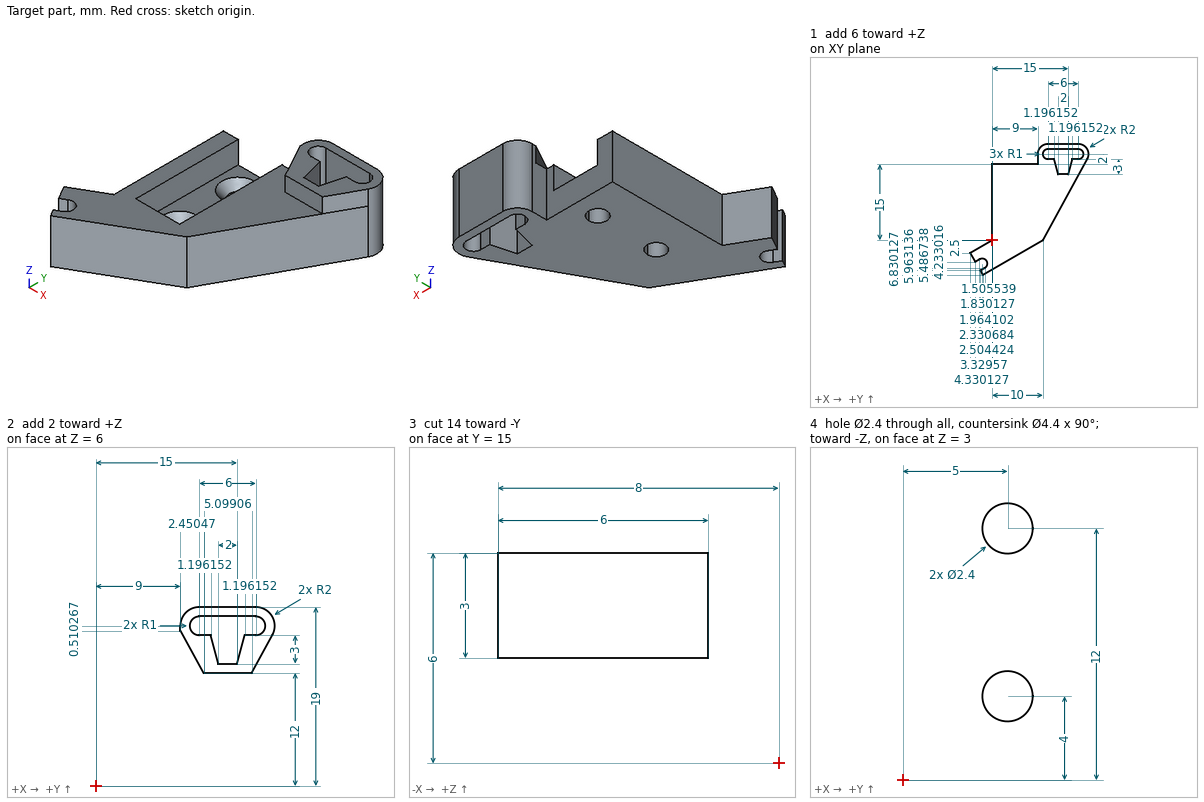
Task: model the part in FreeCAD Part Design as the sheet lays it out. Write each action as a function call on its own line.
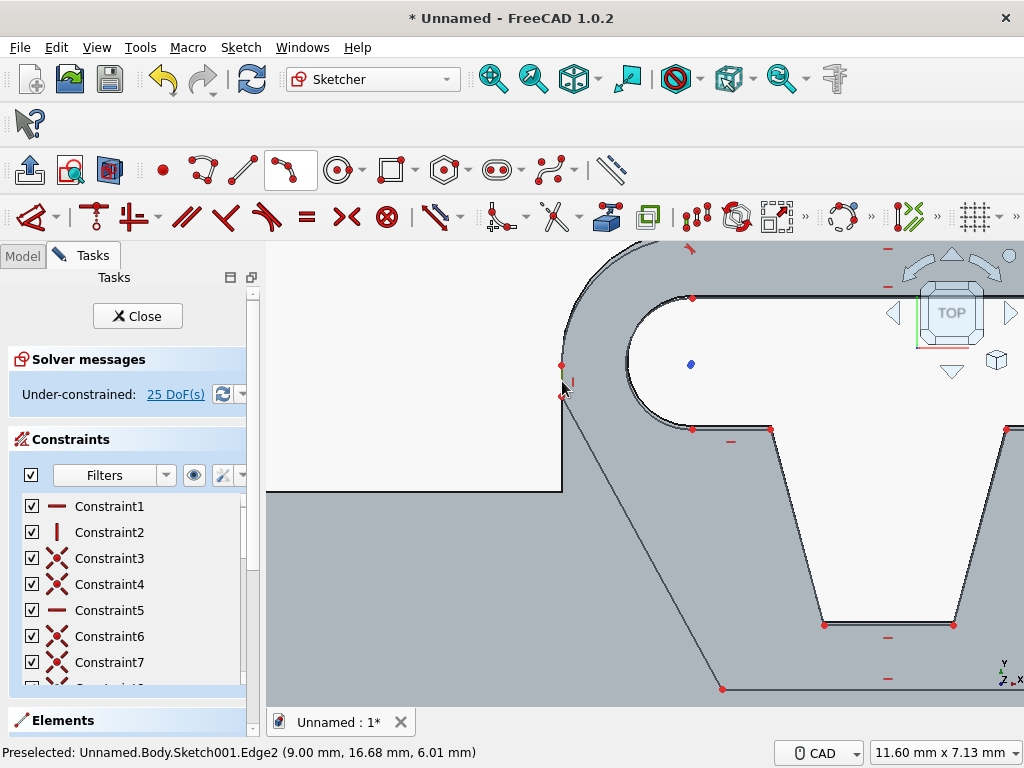
scroll(573, 351, down, 7)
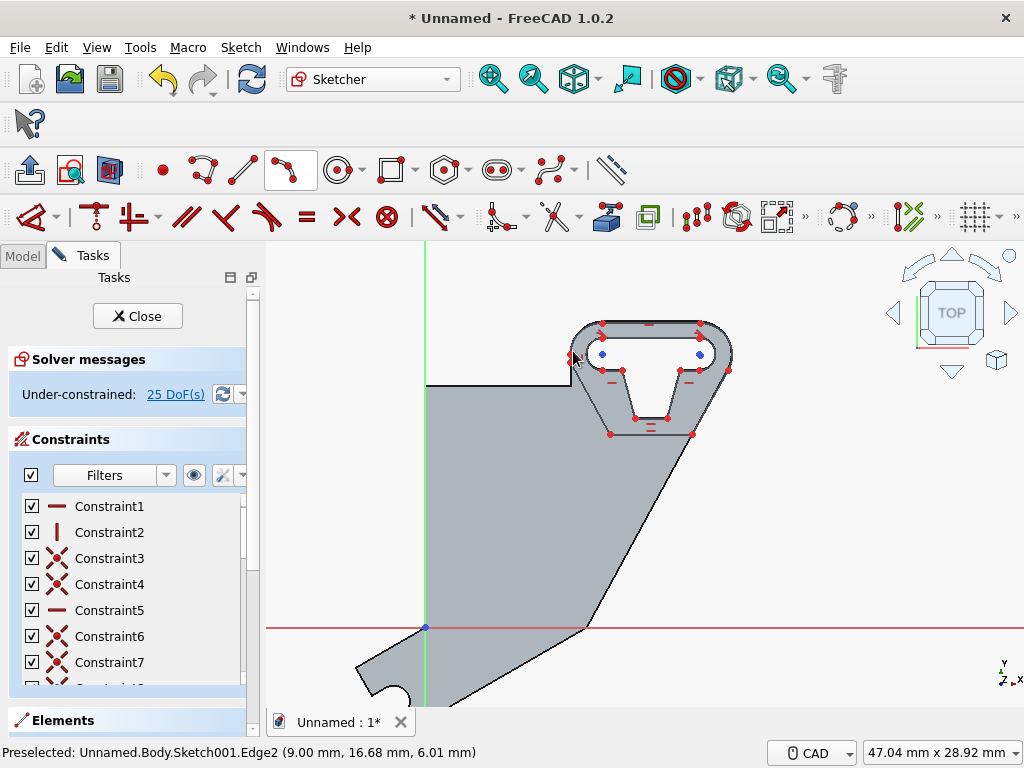
click(574, 340)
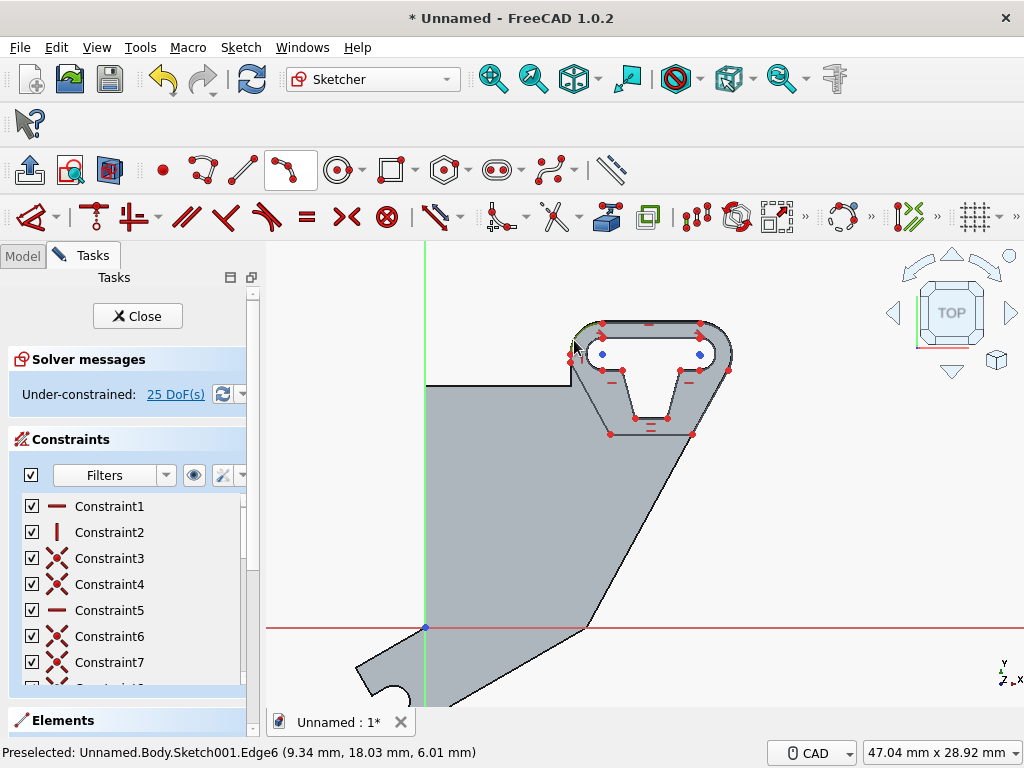
key(t)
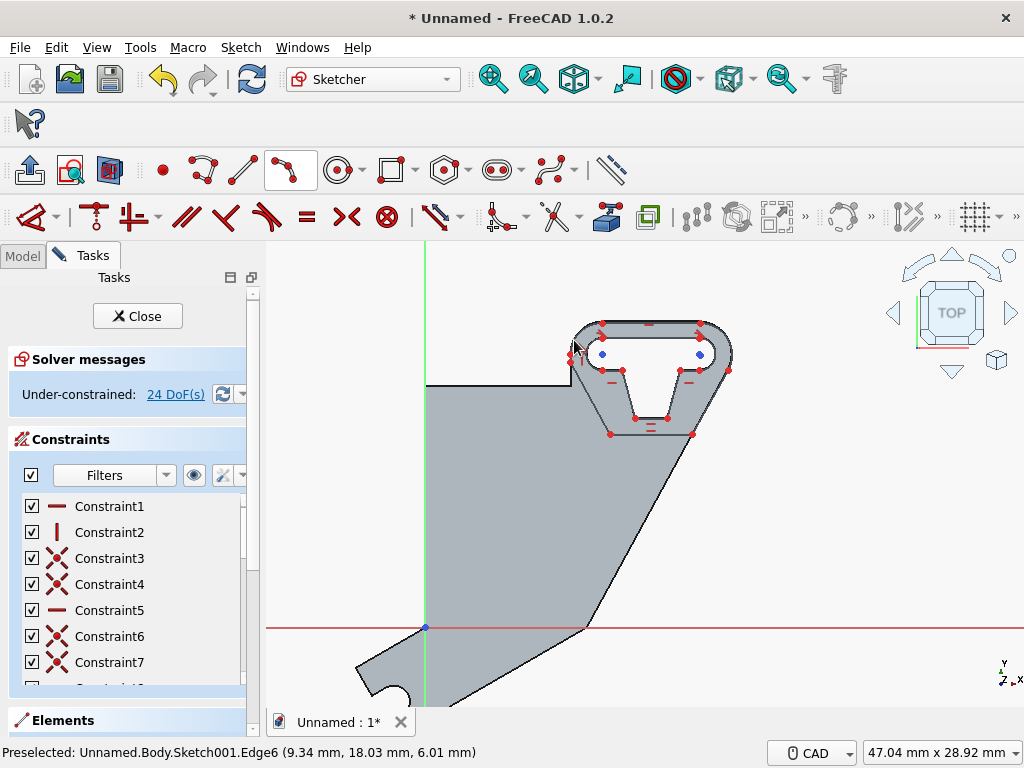
click(703, 415)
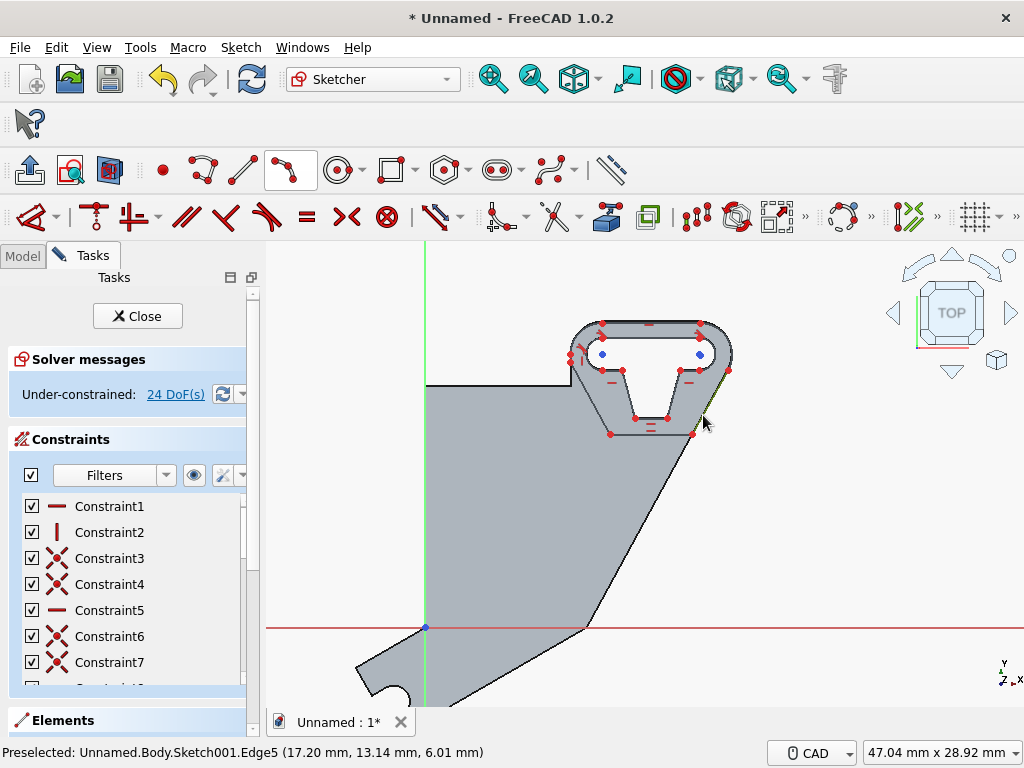
click(732, 351)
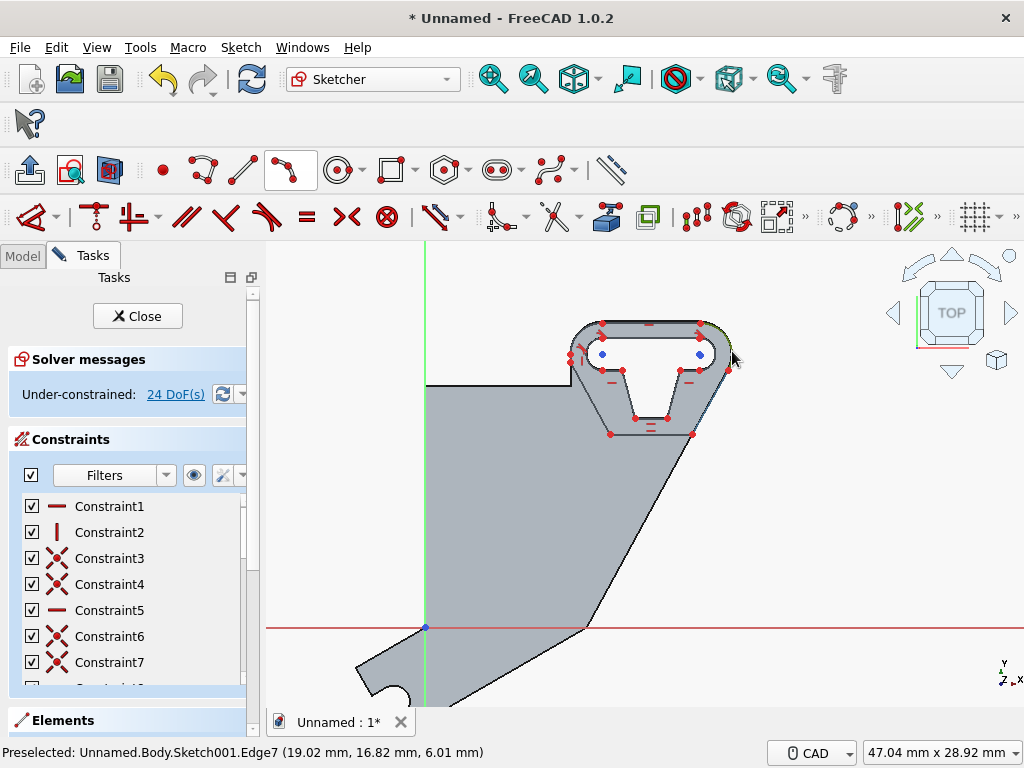
key(t)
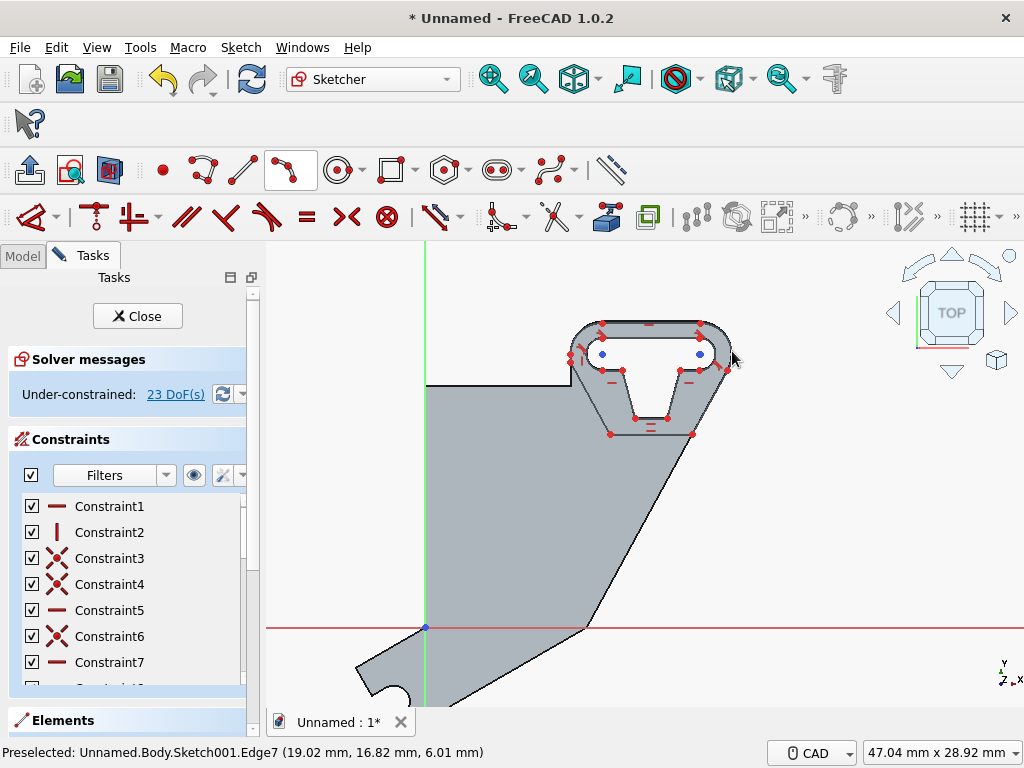
click(632, 338)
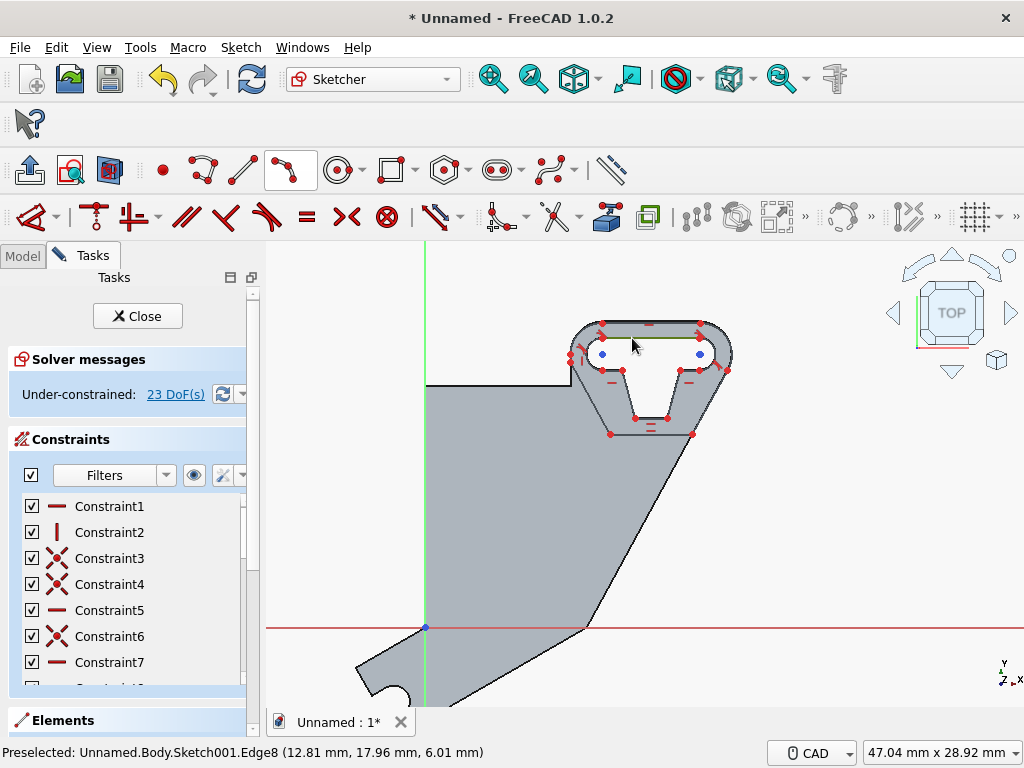
click(712, 345)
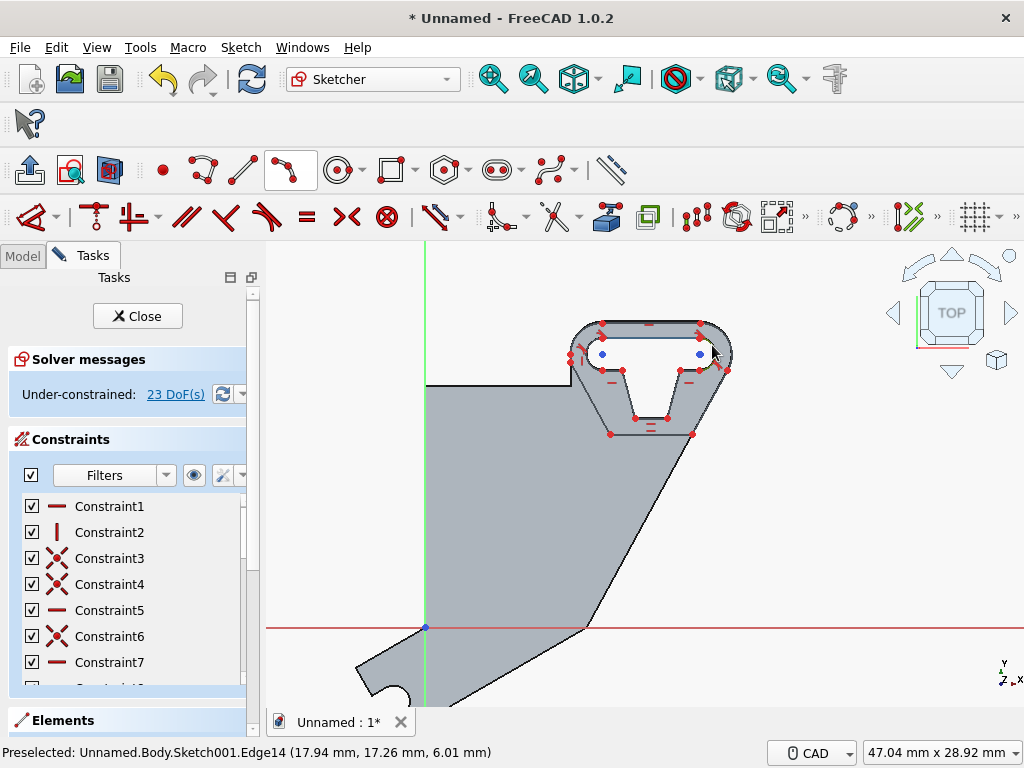
key(t)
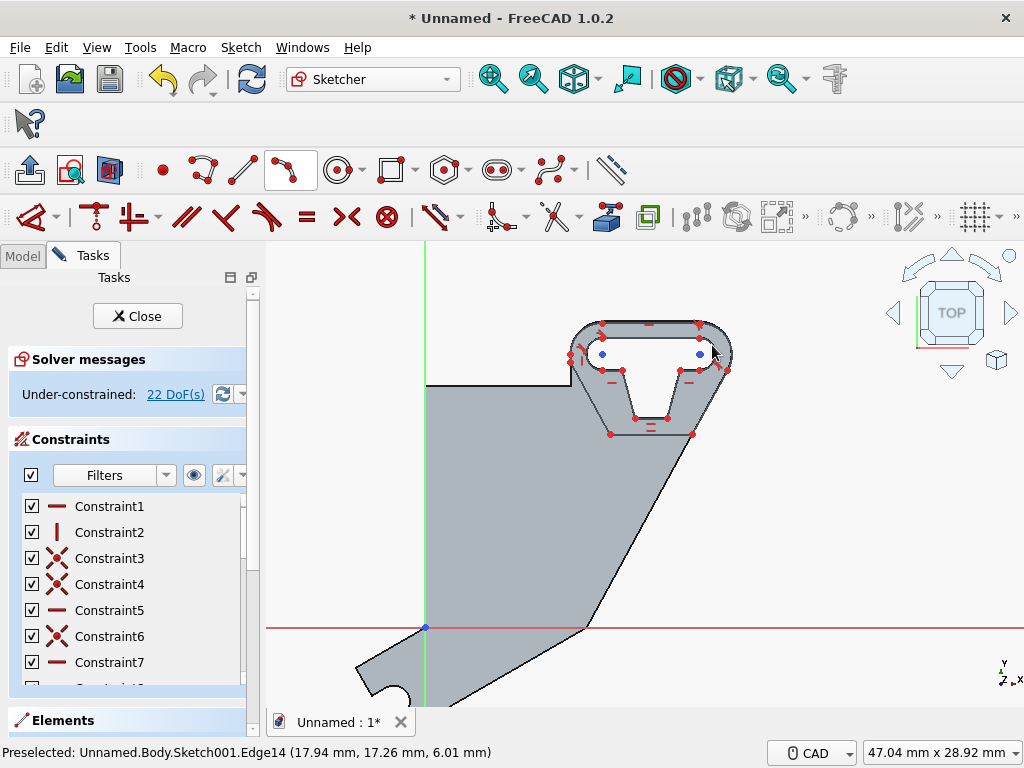
click(632, 338)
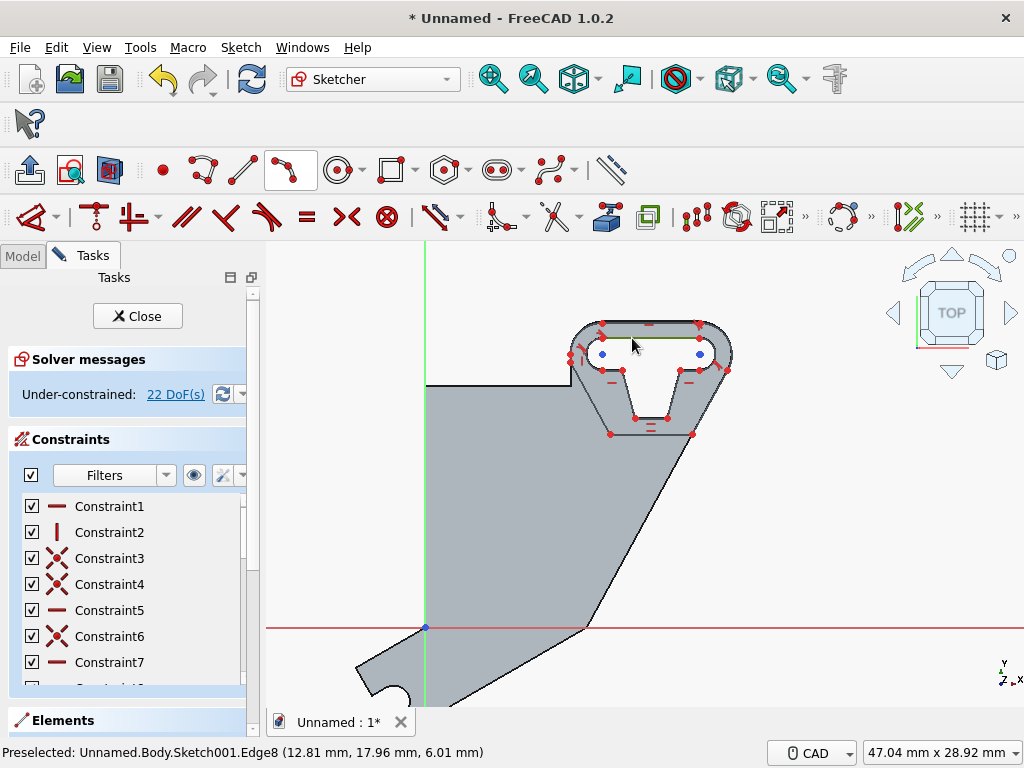
click(590, 345)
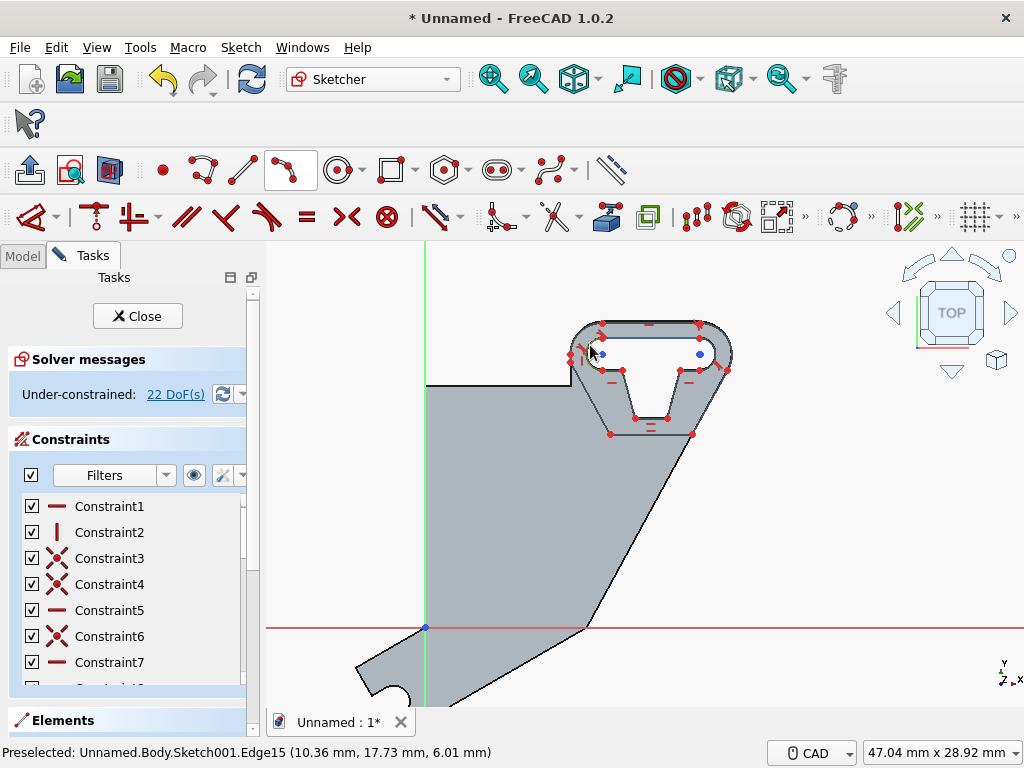
key(t)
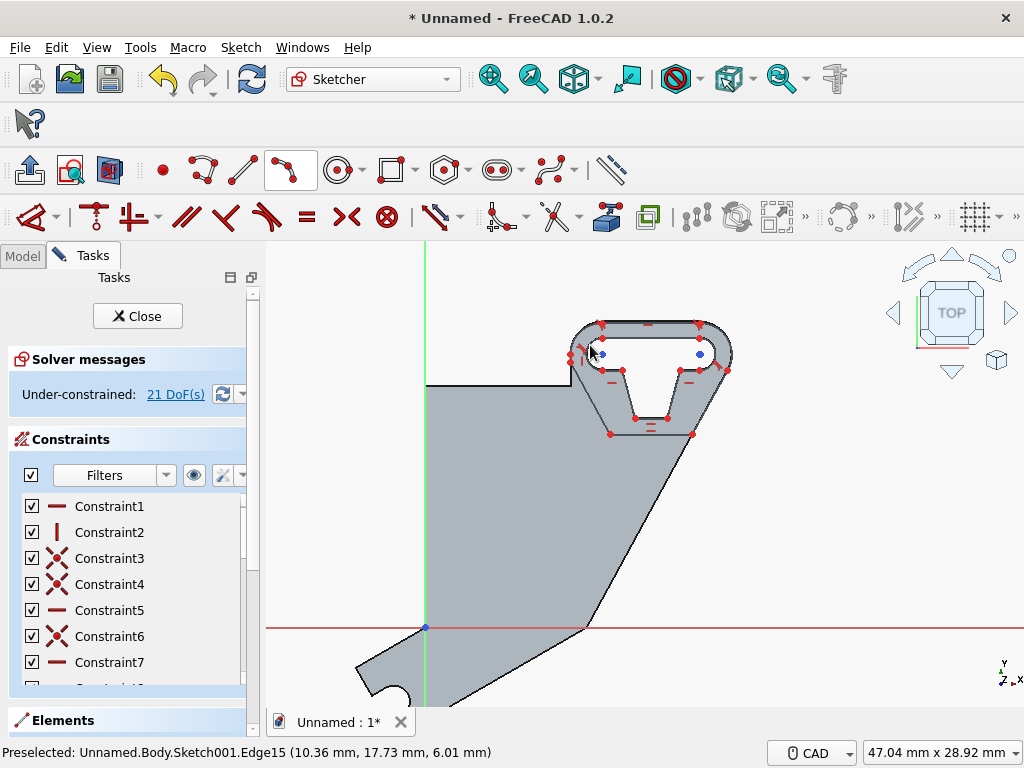
scroll(690, 371, up, 2)